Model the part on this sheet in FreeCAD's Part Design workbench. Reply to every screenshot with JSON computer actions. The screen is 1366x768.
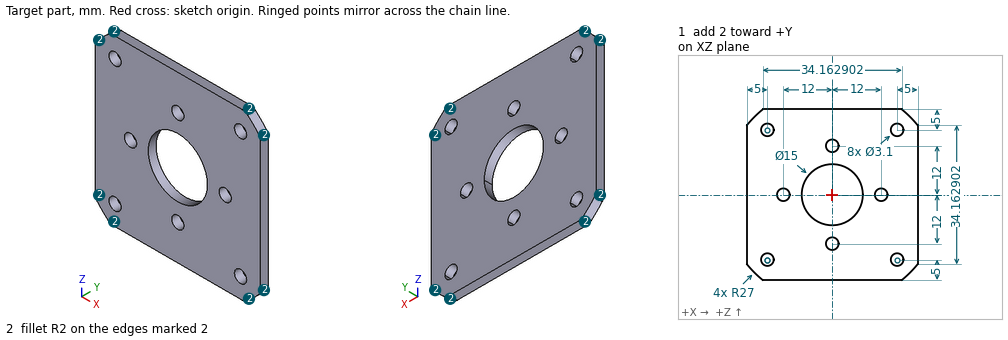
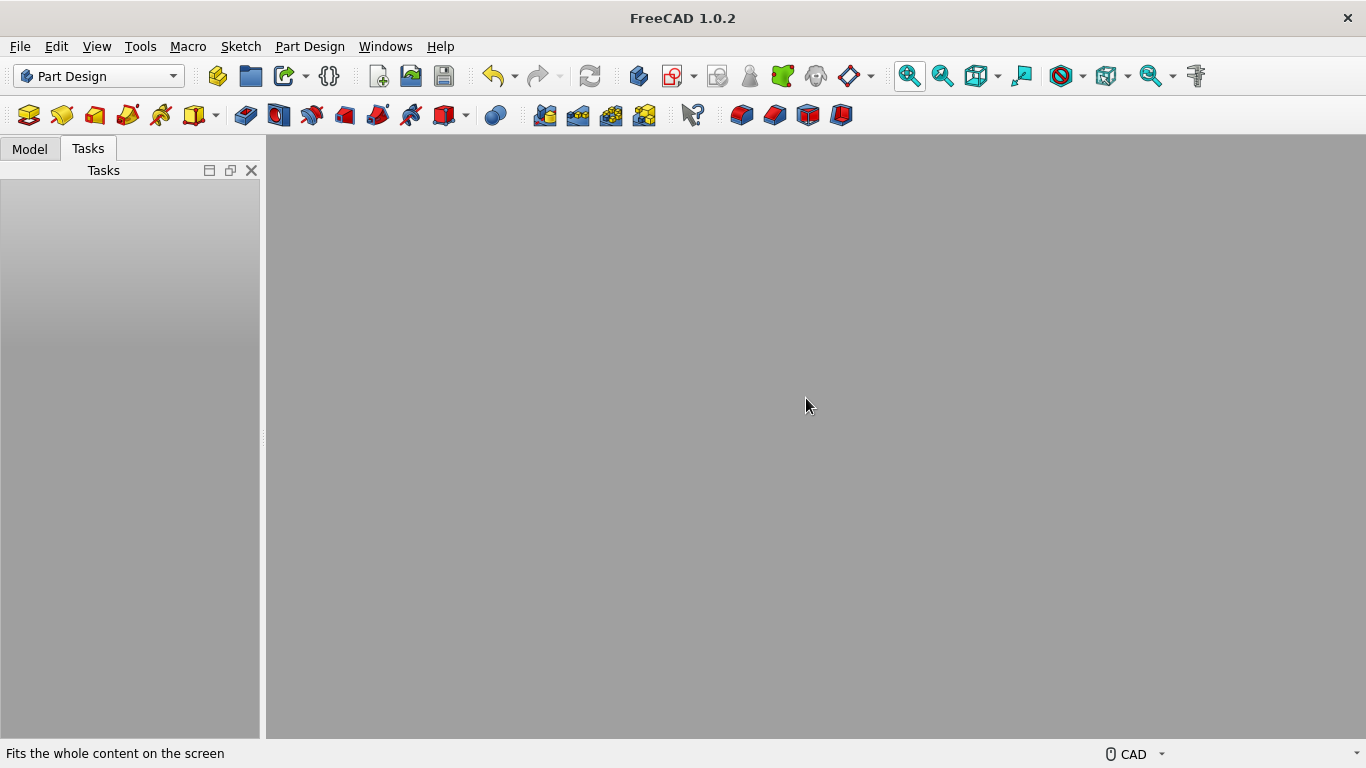
{"action": "left_click", "coordinate": [378, 76]}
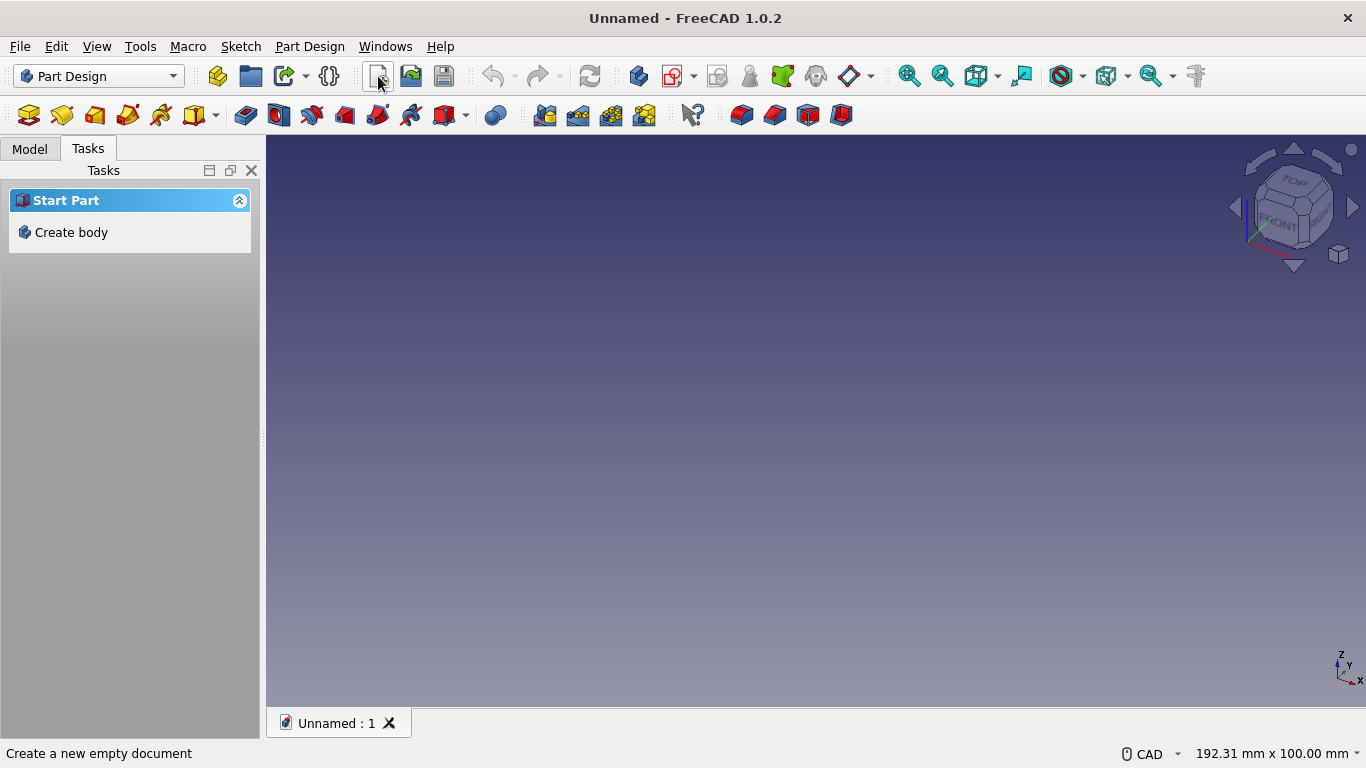
{"action": "left_click", "coordinate": [672, 76]}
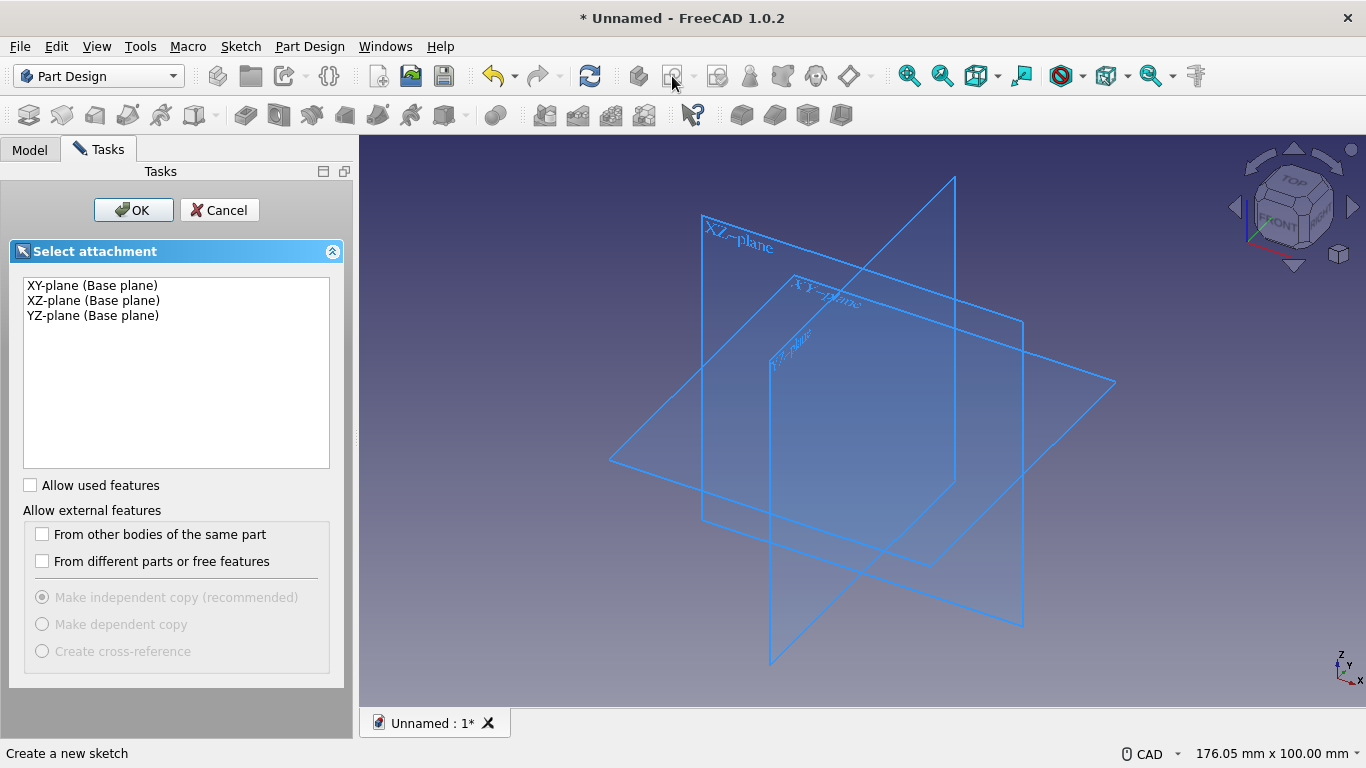
{"action": "left_click", "coordinate": [84, 300]}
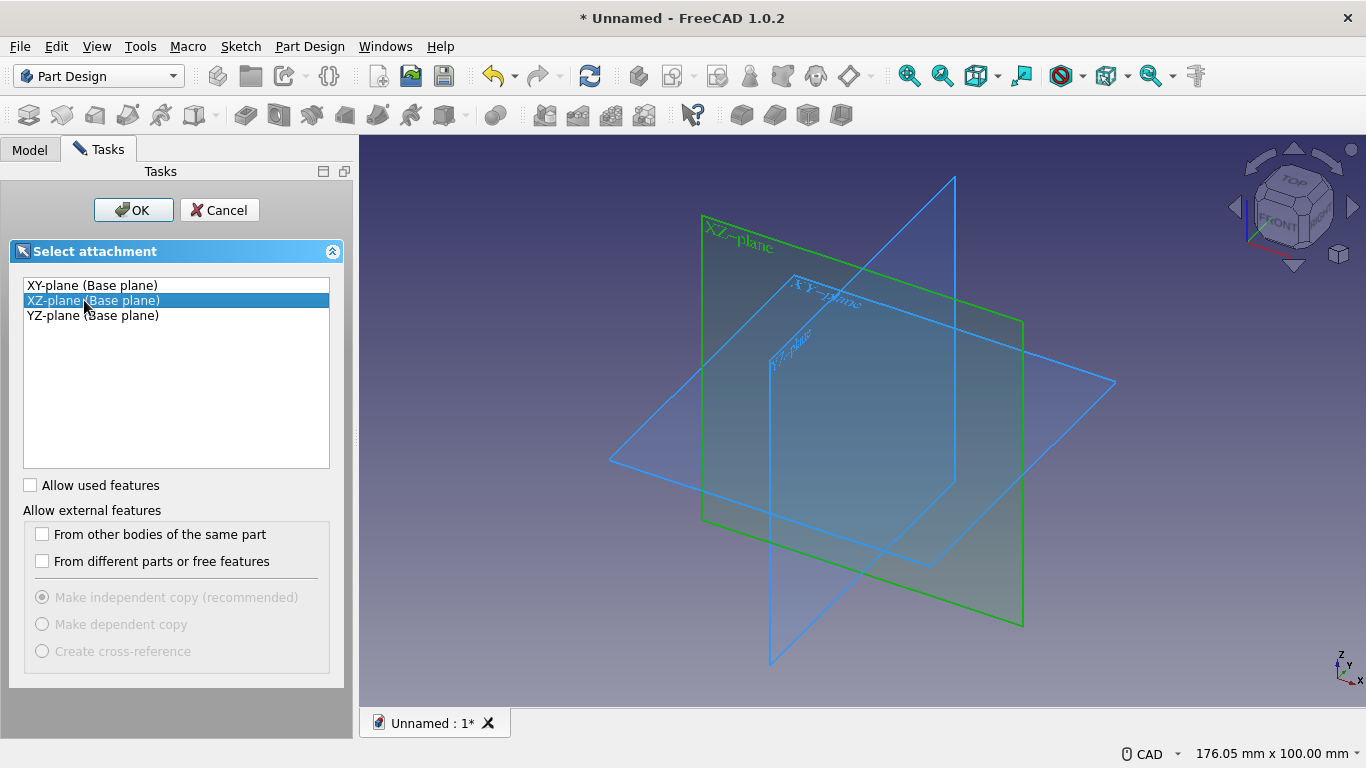
{"action": "left_click", "coordinate": [134, 210]}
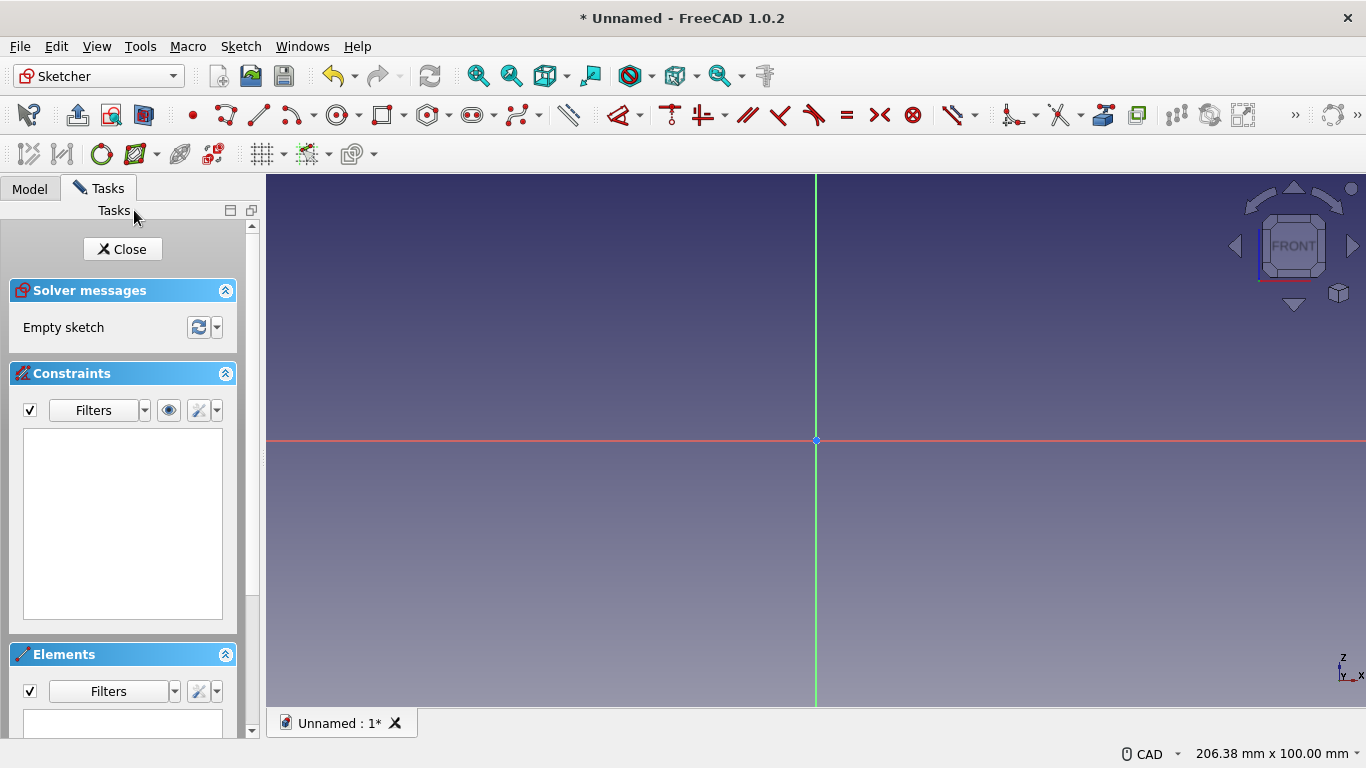
{"action": "scroll", "coordinate": [955, 440], "scroll_direction": "up", "scroll_amount": 2}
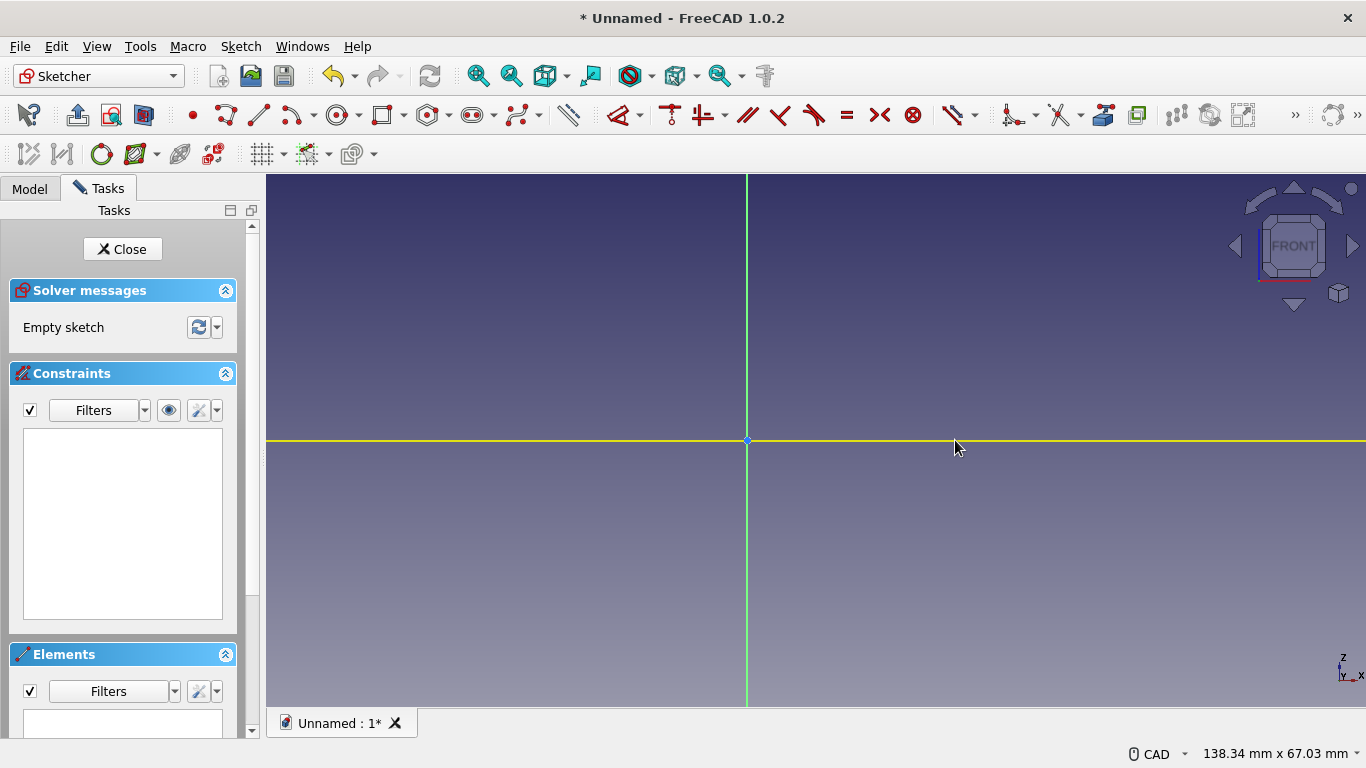
{"action": "left_click", "coordinate": [259, 116]}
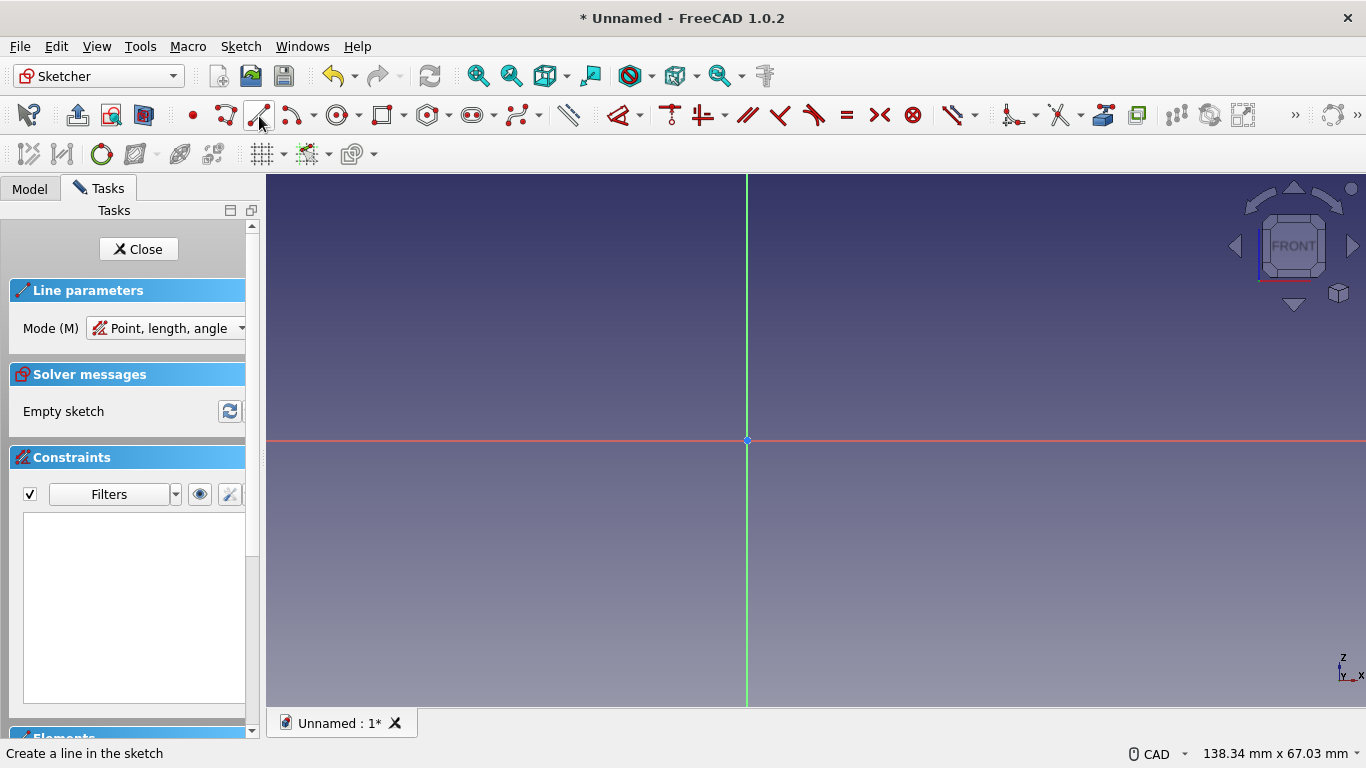
{"action": "left_click", "coordinate": [612, 274]}
{"action": "left_click", "coordinate": [883, 274]}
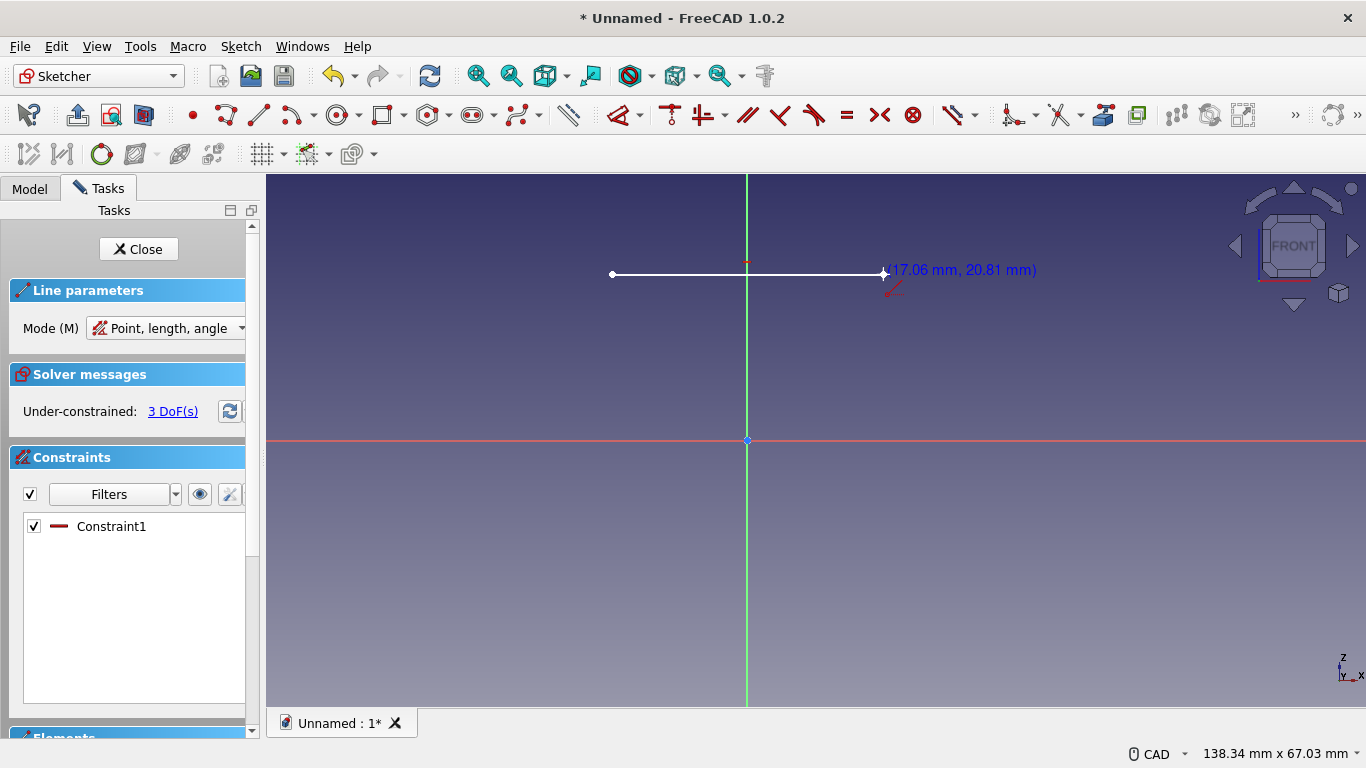
{"action": "left_click", "coordinate": [914, 305]}
{"action": "left_click", "coordinate": [914, 576]}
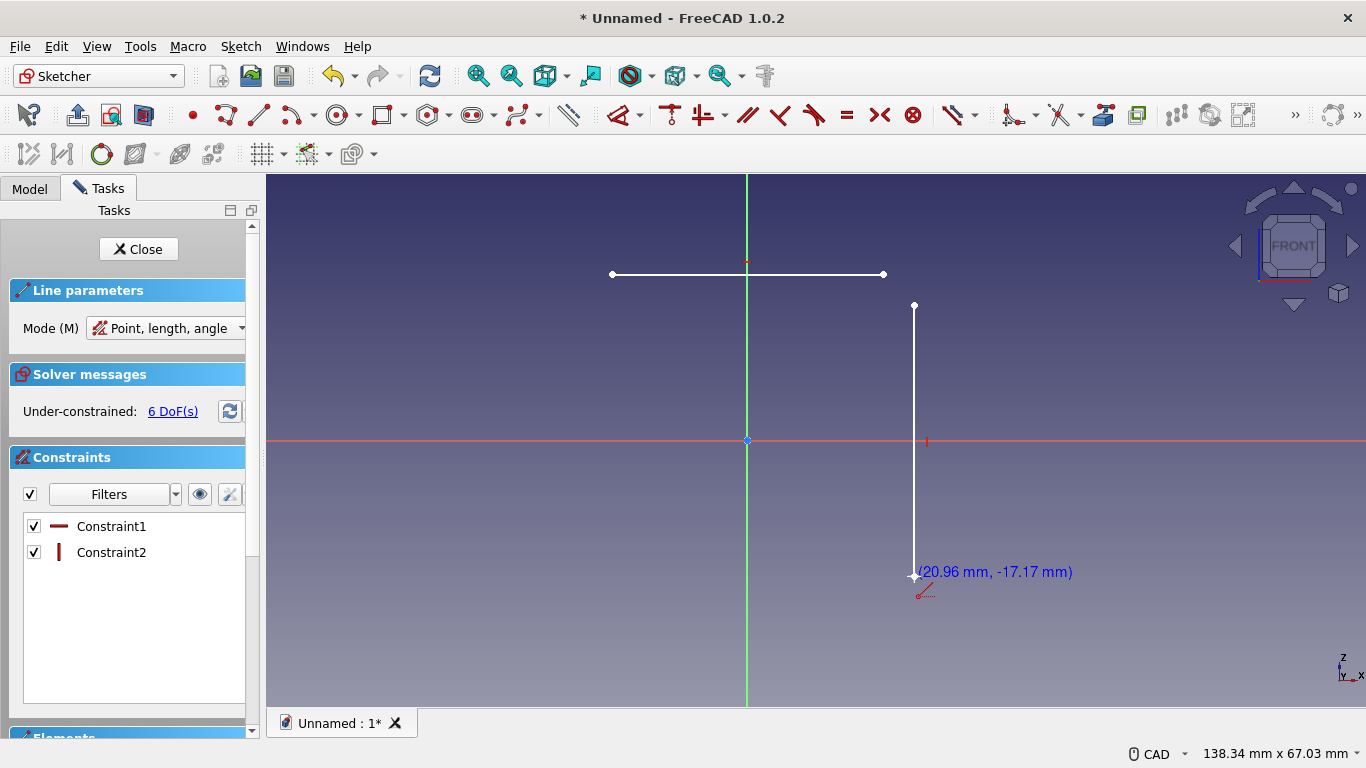
{"action": "left_click", "coordinate": [883, 607]}
{"action": "left_click", "coordinate": [612, 607]}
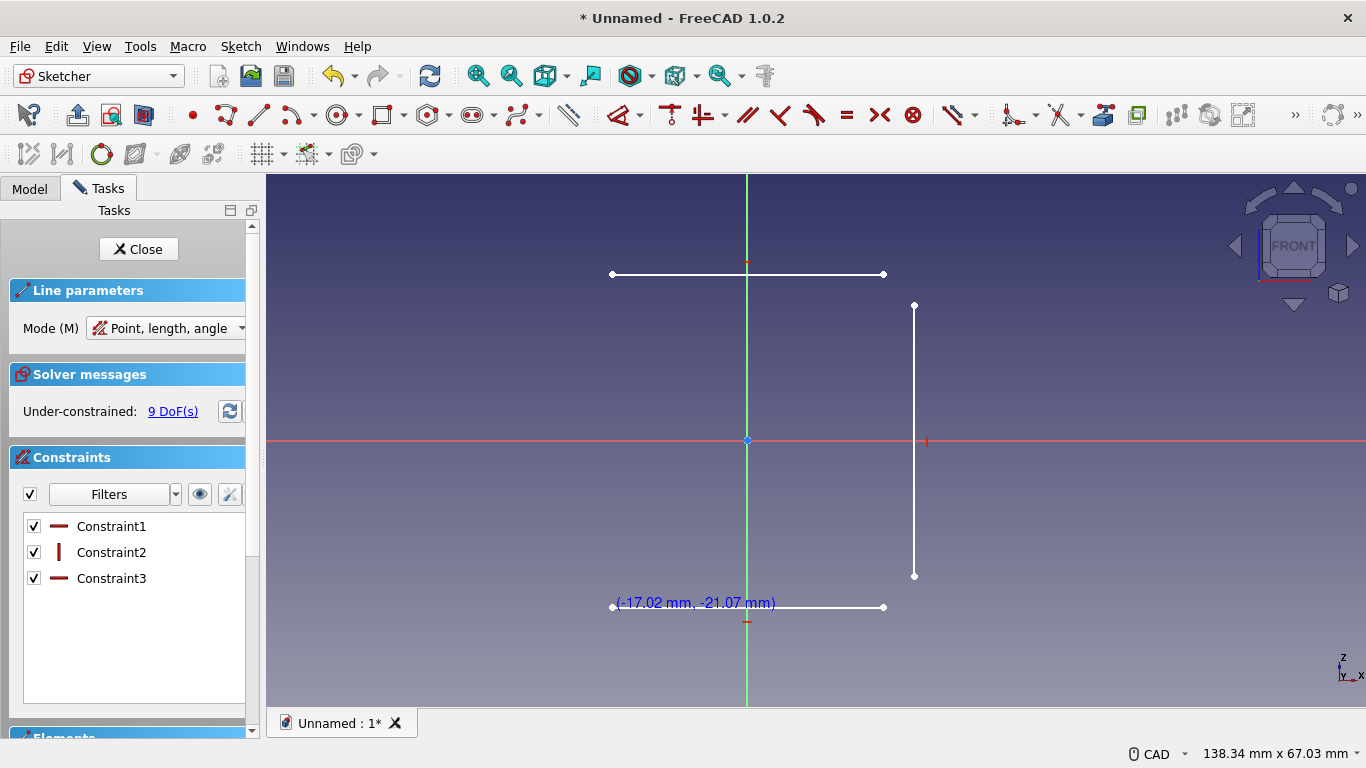
{"action": "left_click", "coordinate": [581, 576]}
{"action": "left_click", "coordinate": [581, 305]}